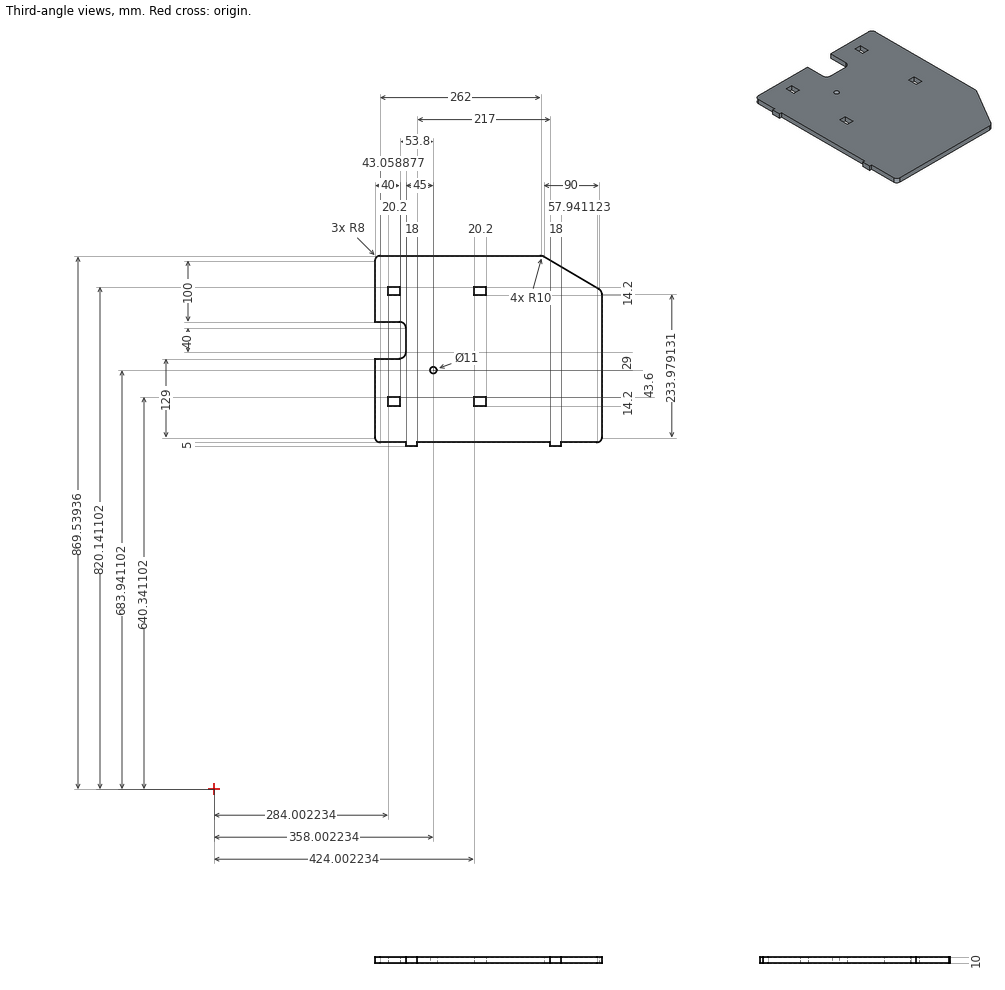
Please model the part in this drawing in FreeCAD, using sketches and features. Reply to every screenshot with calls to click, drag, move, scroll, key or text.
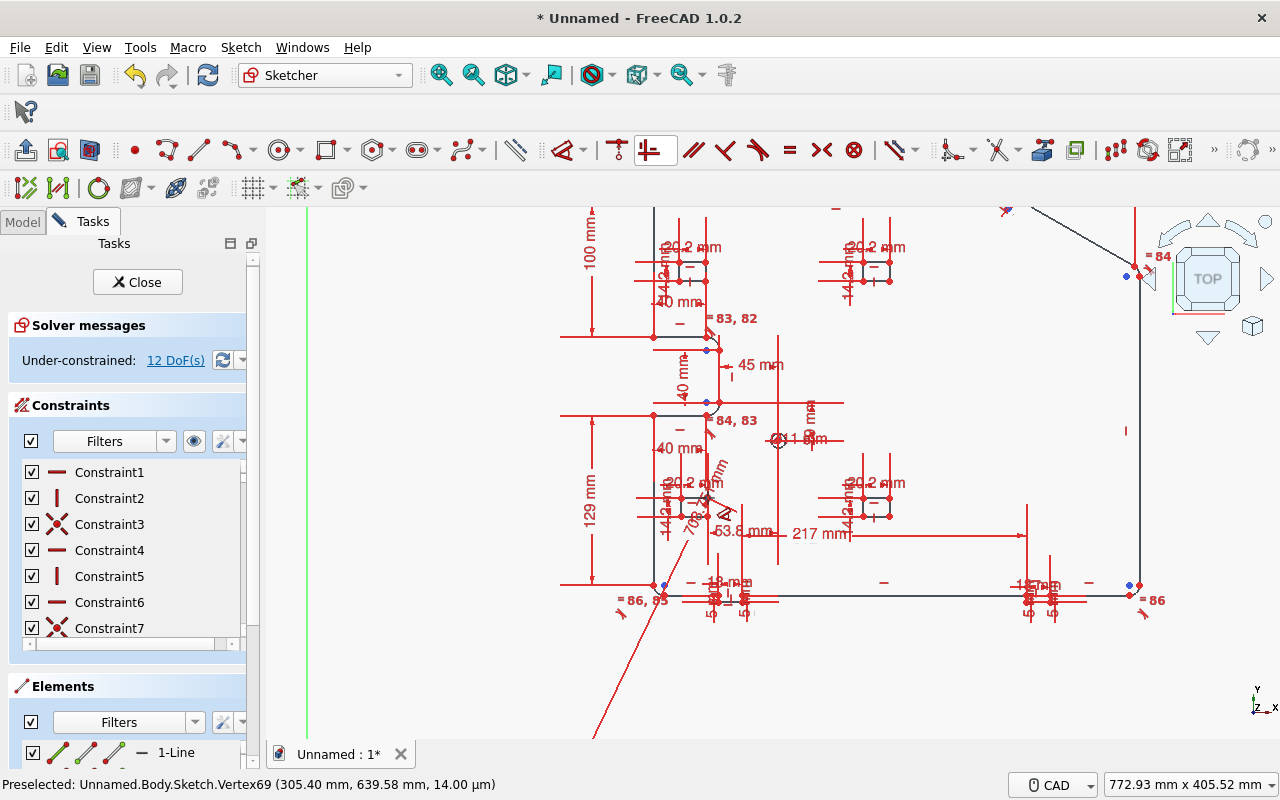
click(778, 441)
click(812, 469)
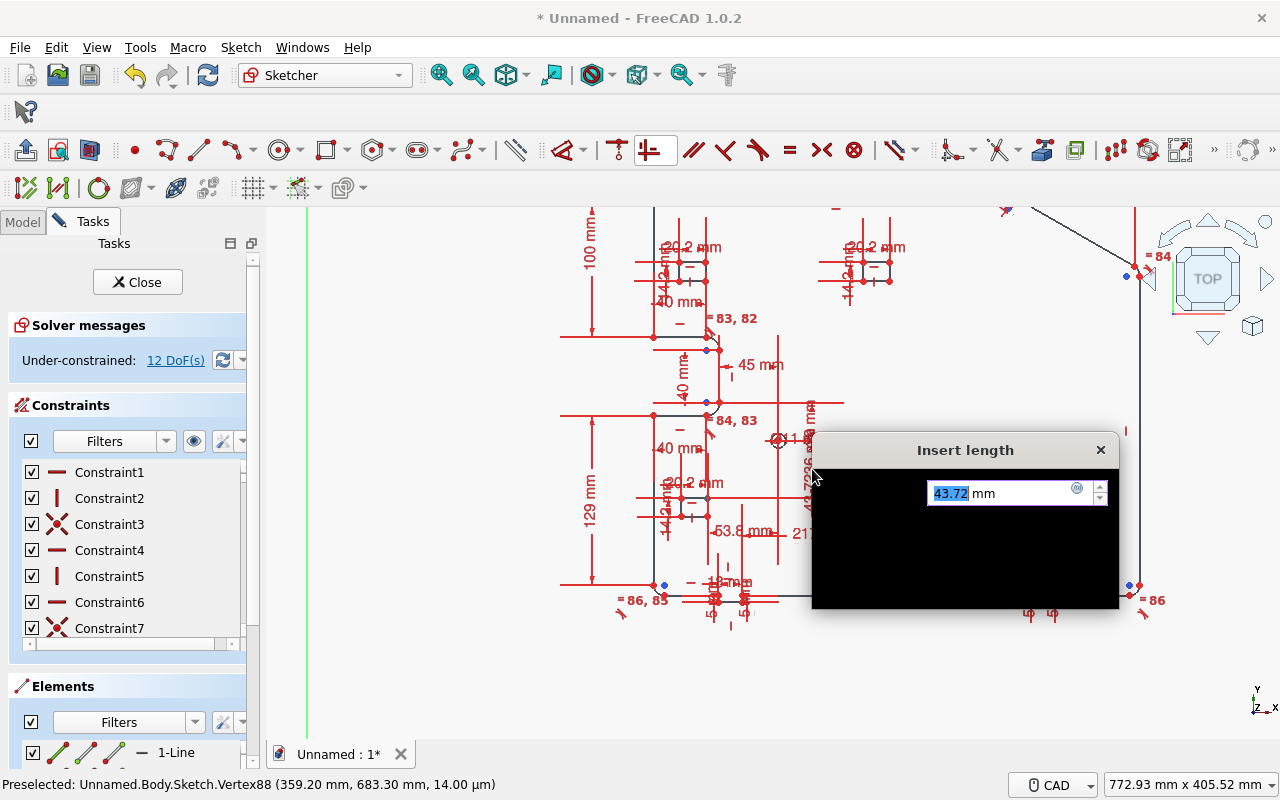
text(43.6)
key(Return)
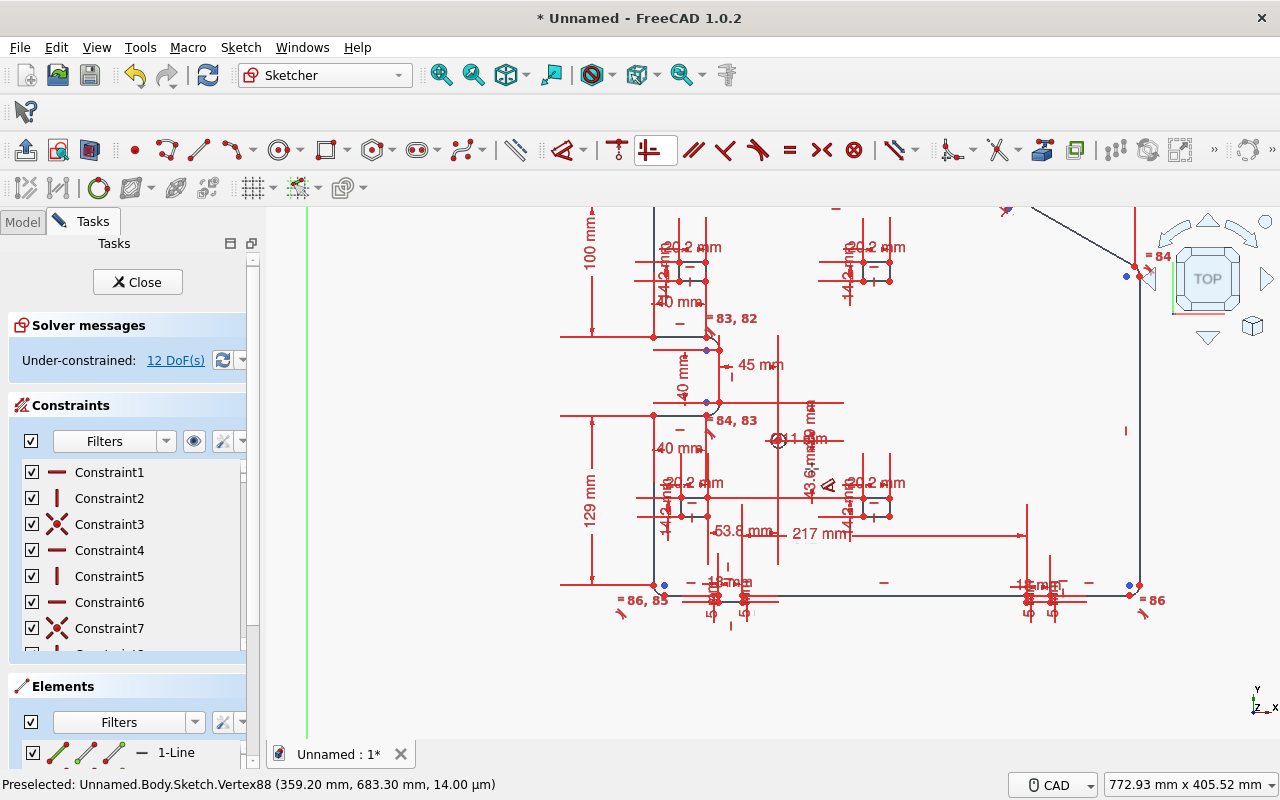
click(681, 596)
click(691, 562)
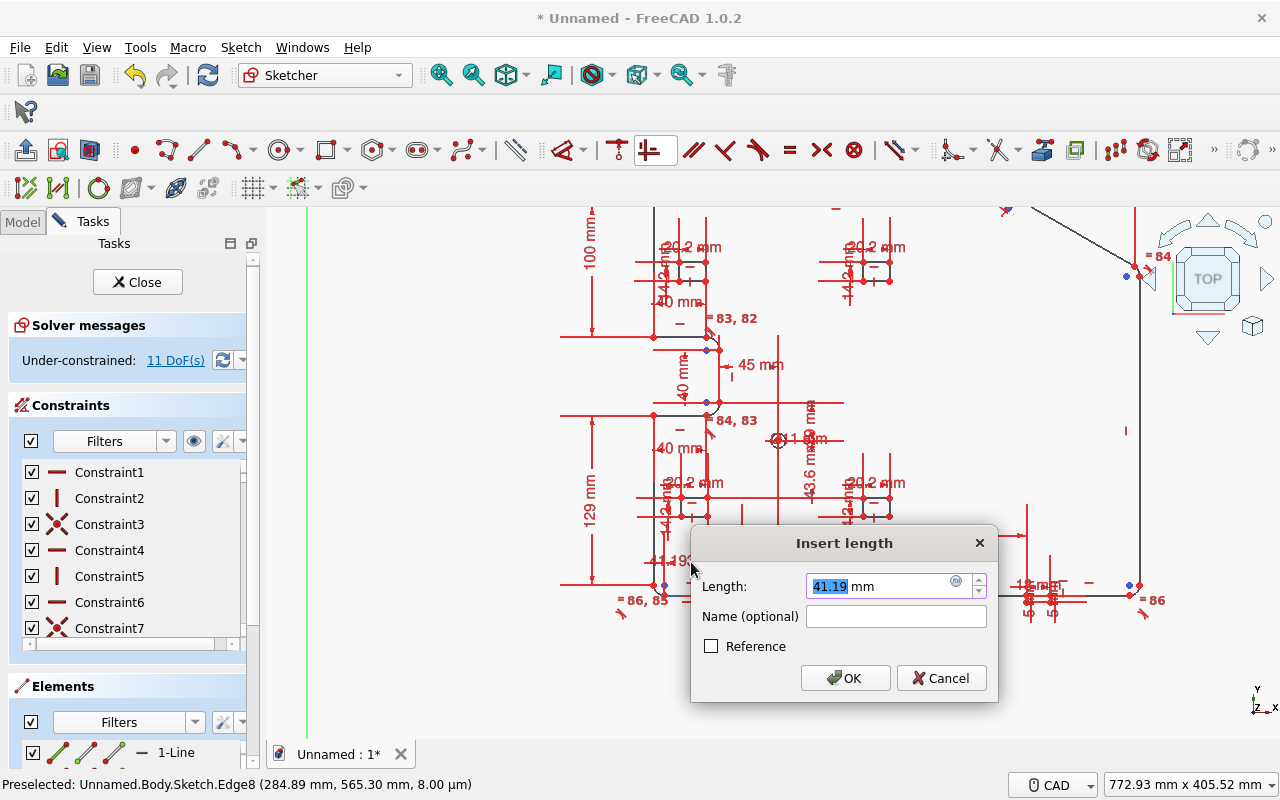
text(43.058877)
key(Return)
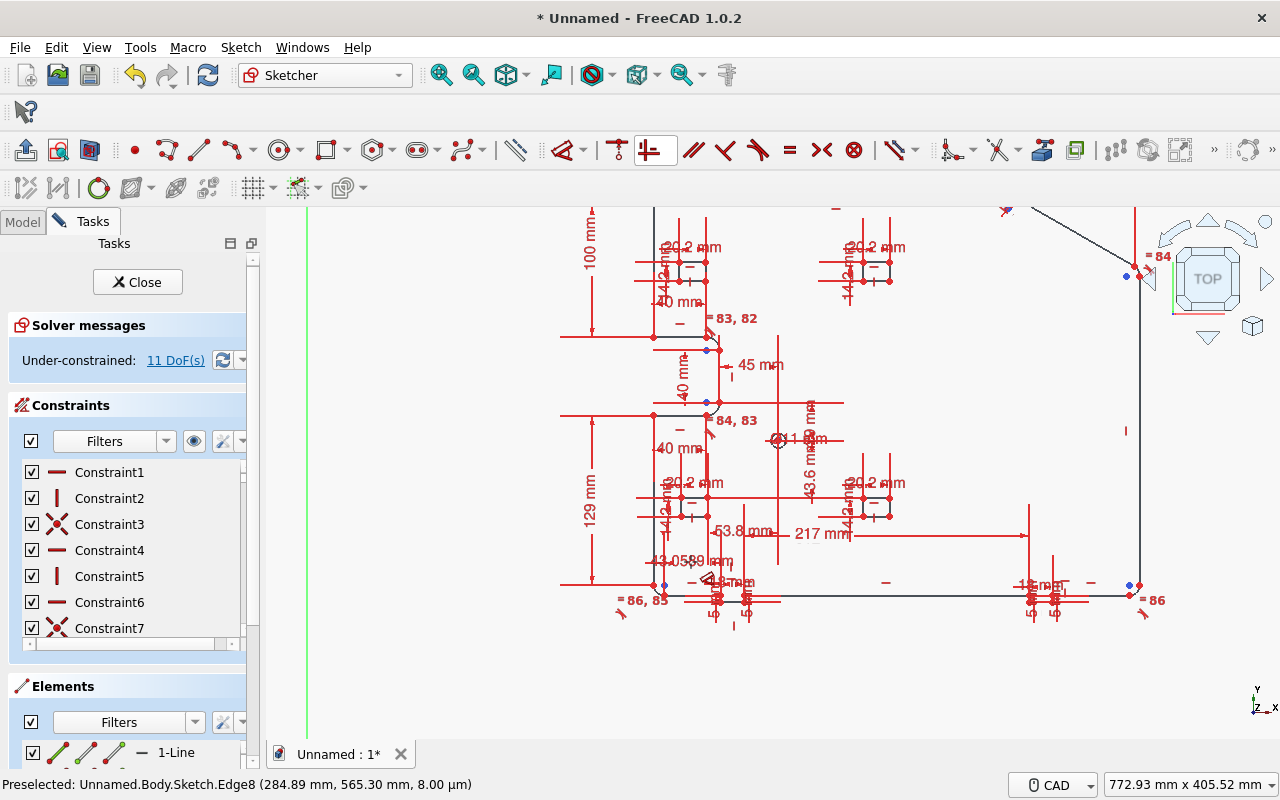
click(1076, 596)
click(1084, 562)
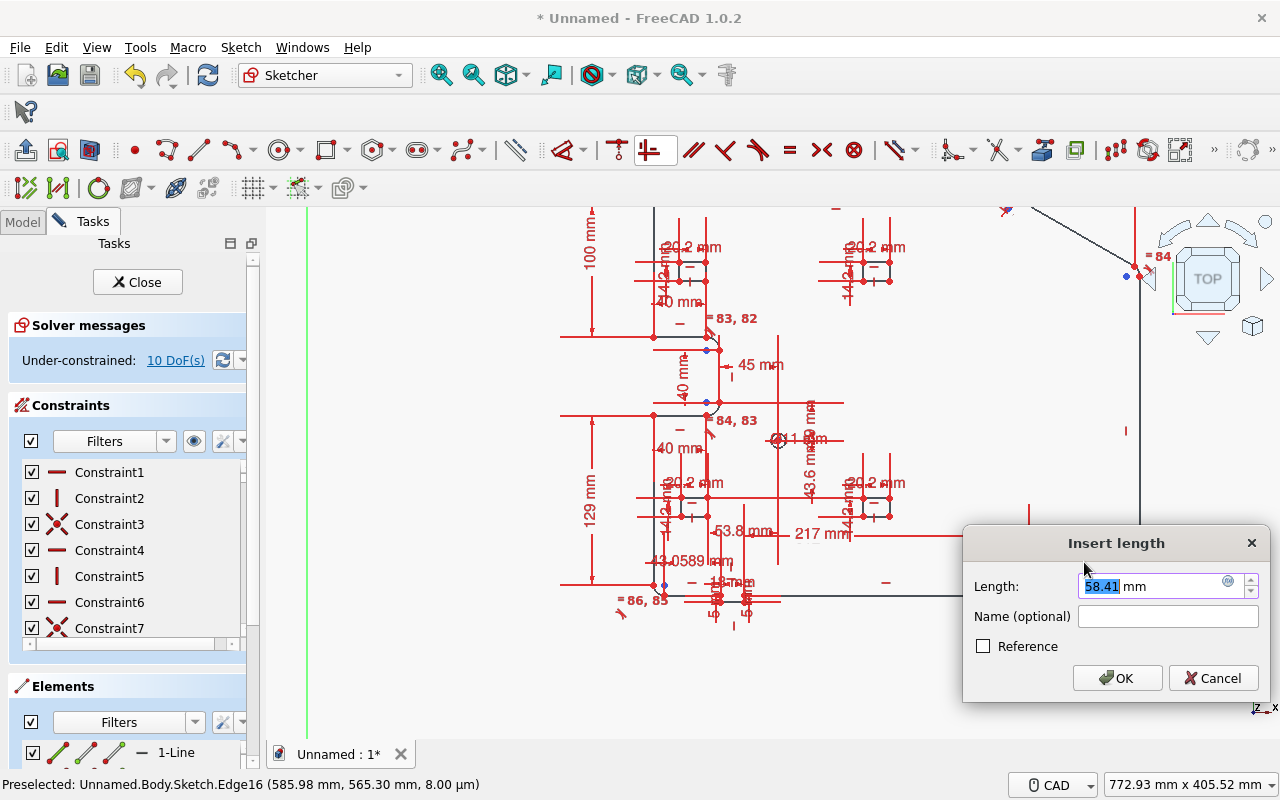
text(57.941123)
key(Return)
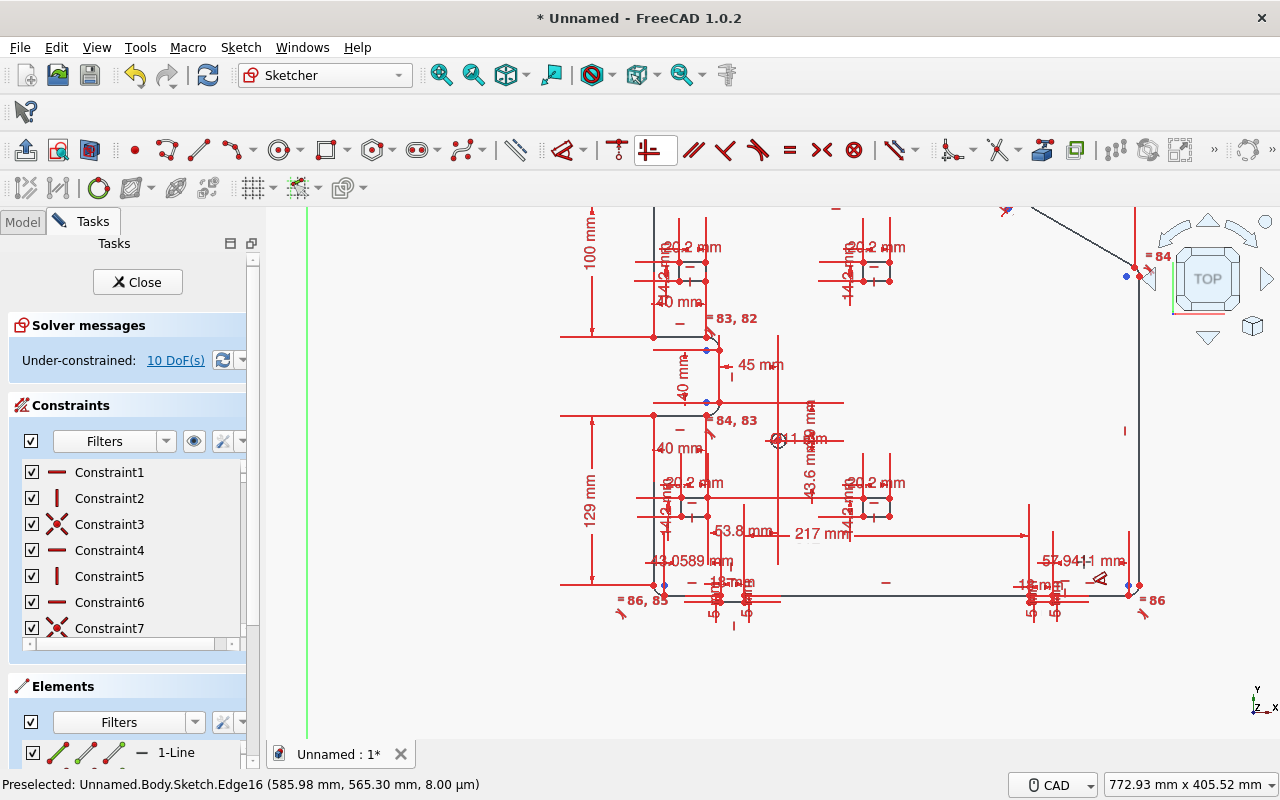
scroll(697, 347, down, 6)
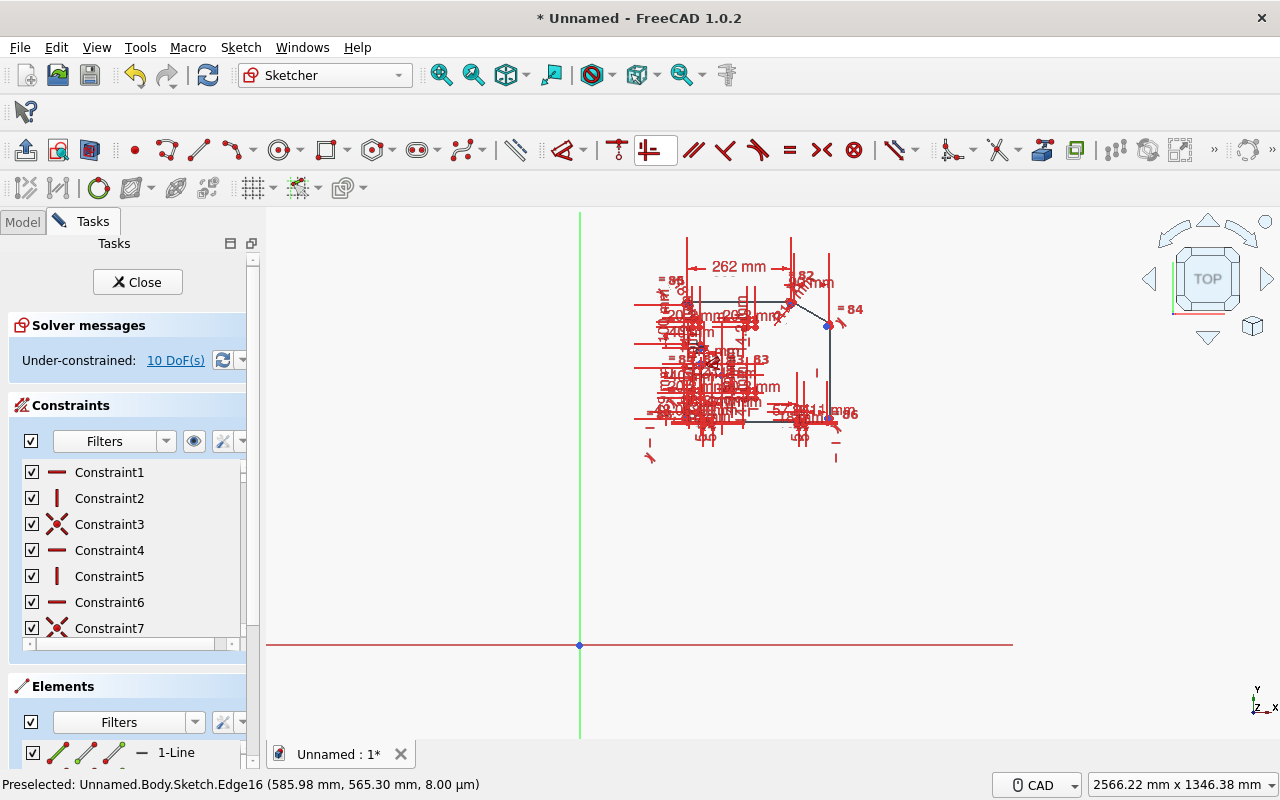
click(831, 391)
click(865, 372)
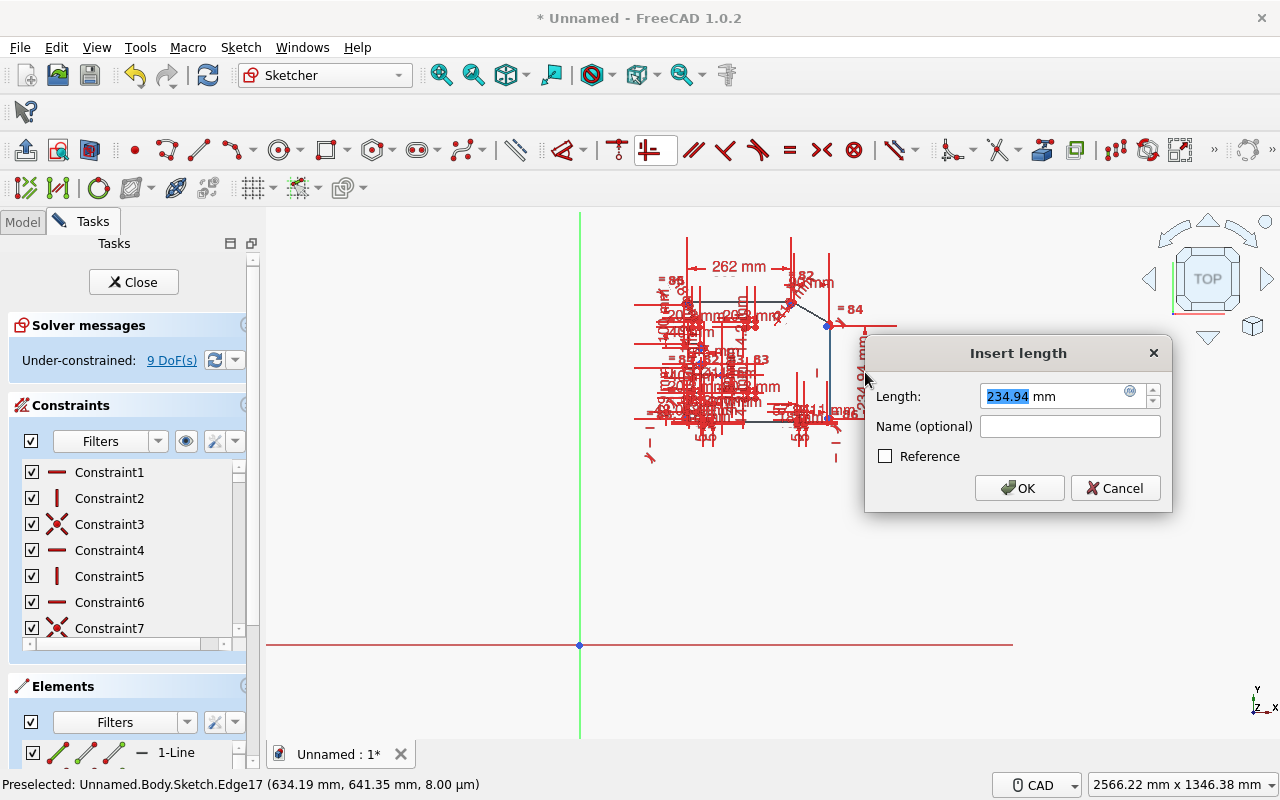
text(233.979131)
key(Return)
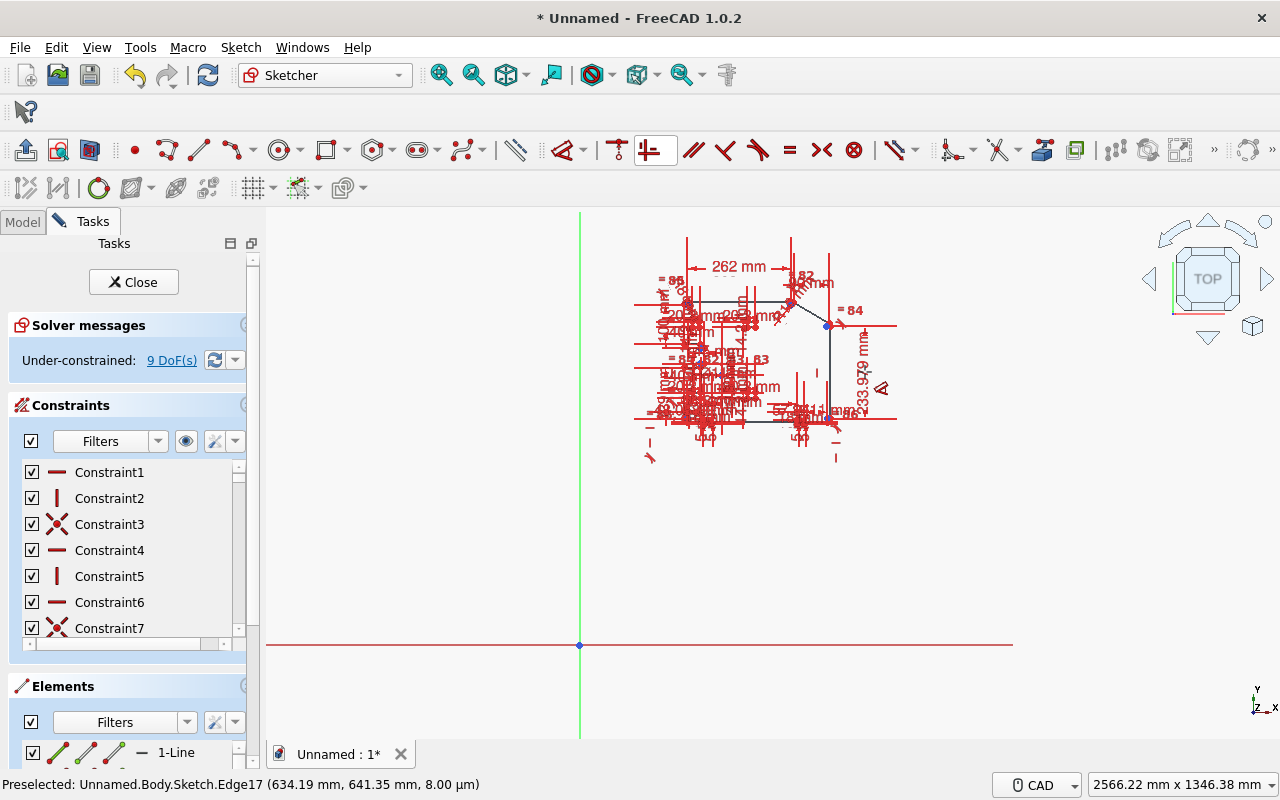
scroll(794, 303, up, 8)